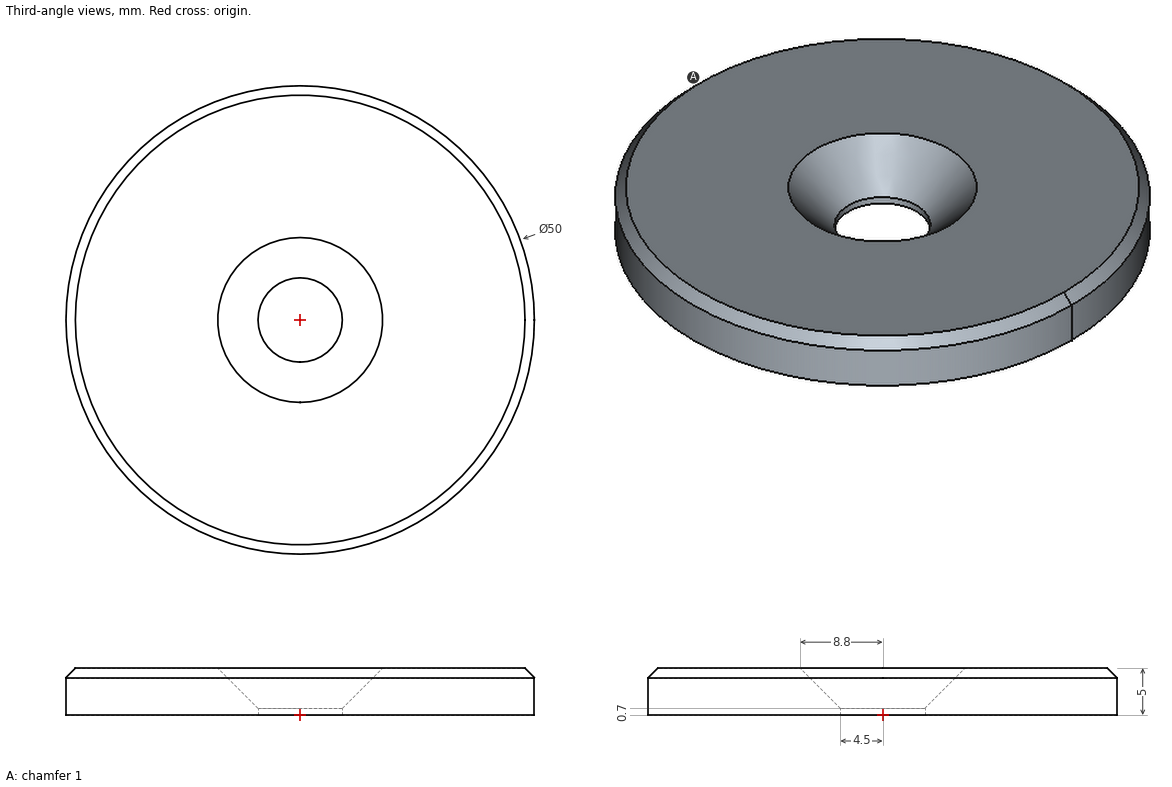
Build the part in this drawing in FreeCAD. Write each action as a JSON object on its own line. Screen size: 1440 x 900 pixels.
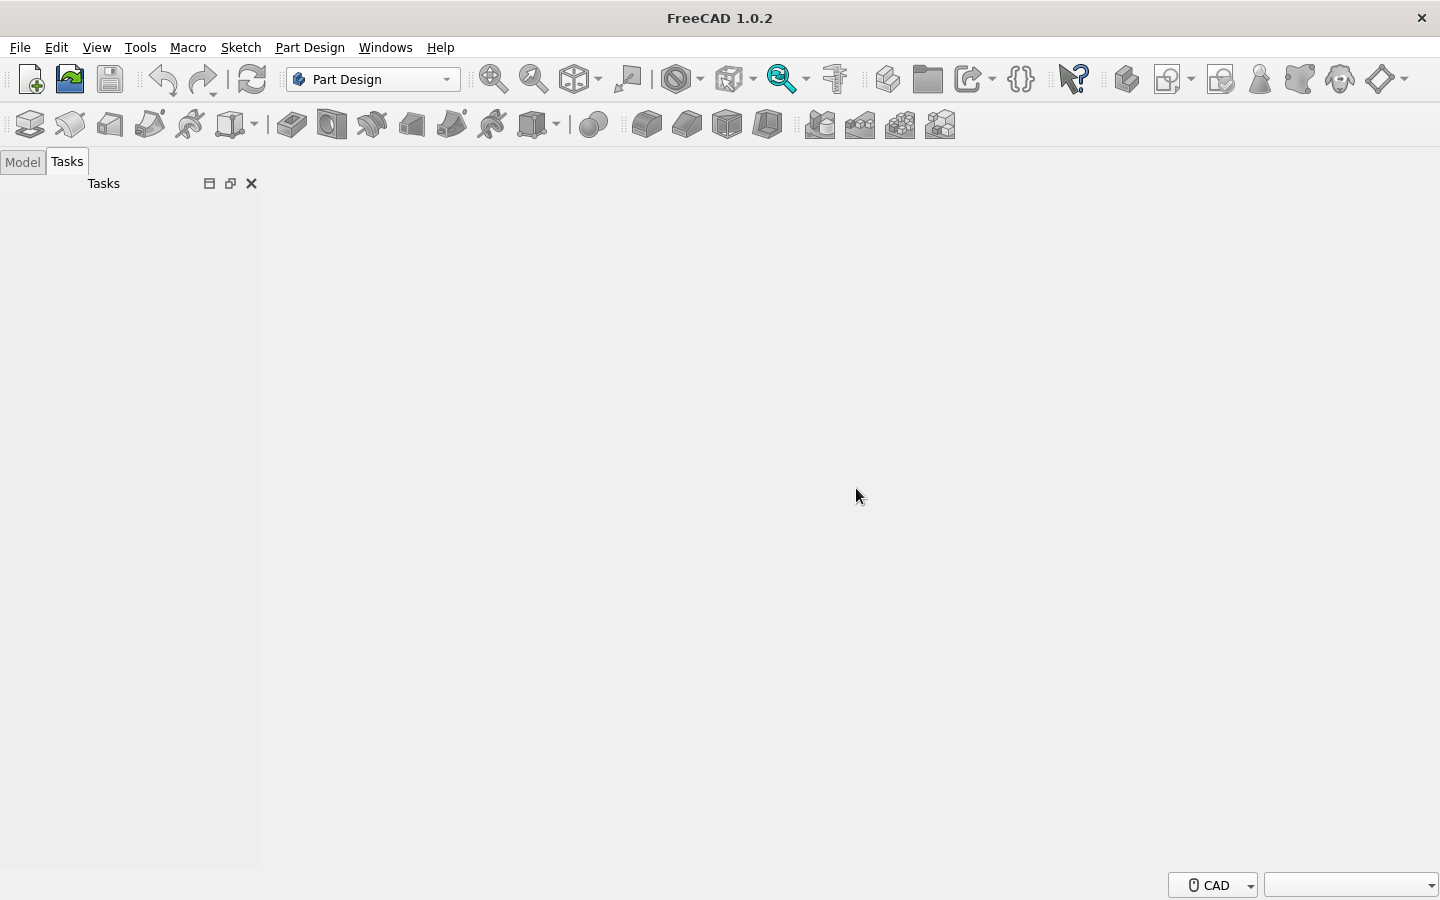
{"action": "left_click", "coordinate": [30, 80]}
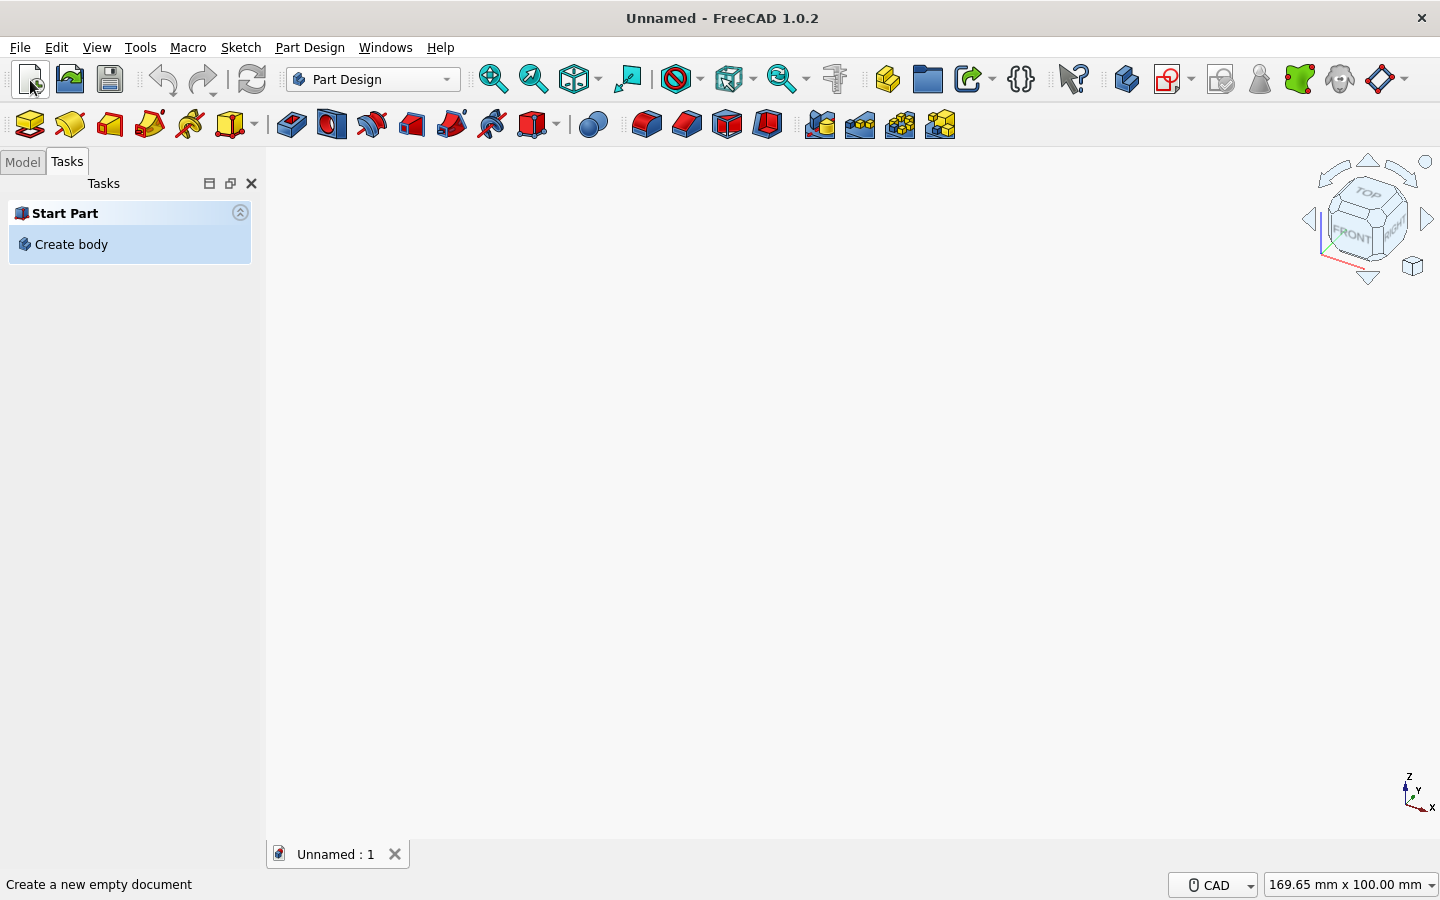
{"action": "left_click", "coordinate": [1168, 80]}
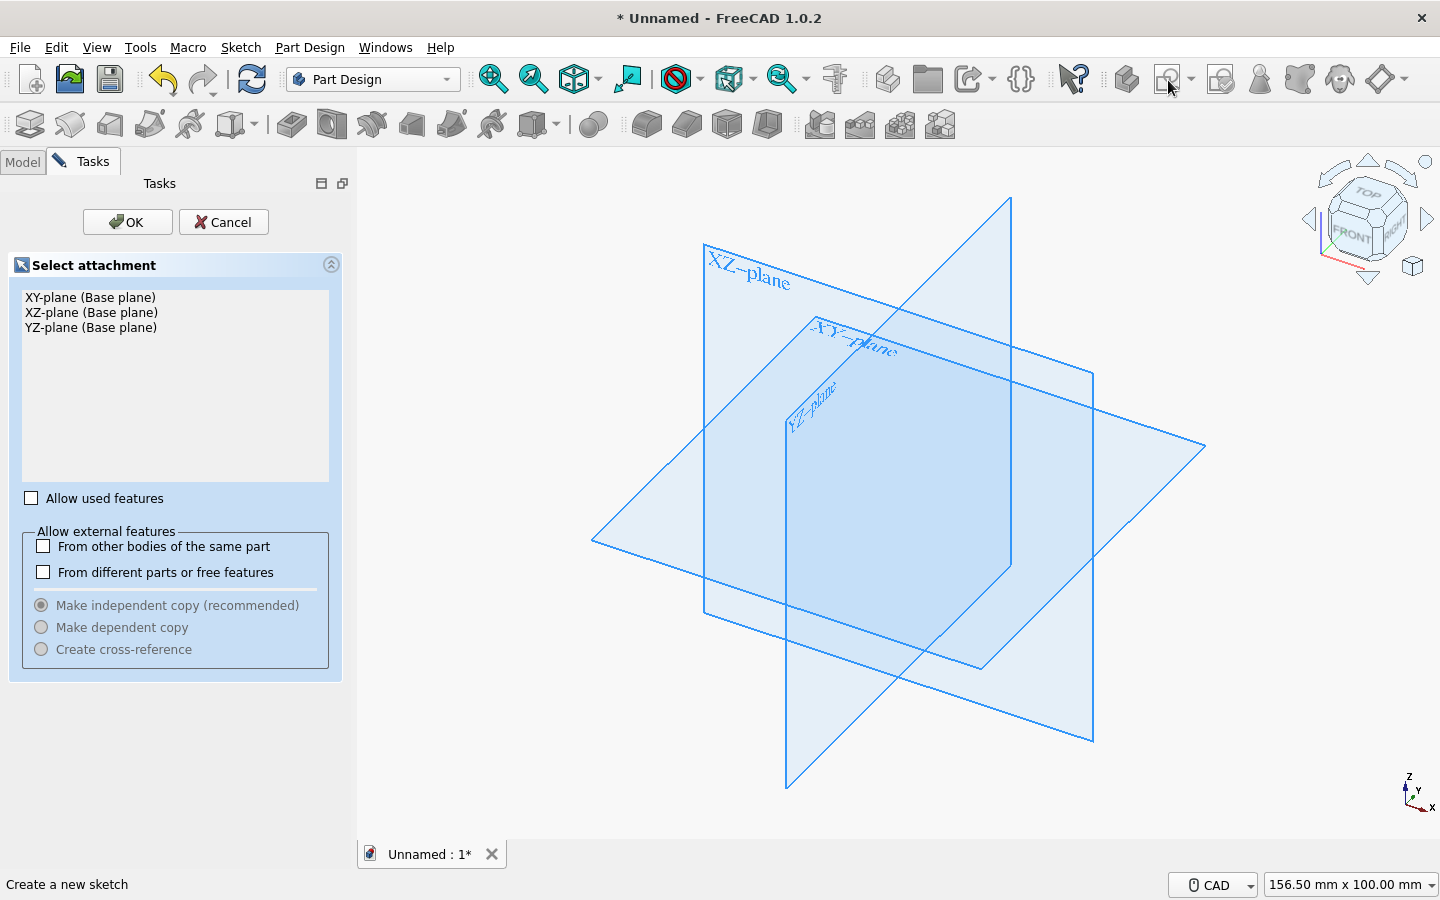
{"action": "left_click", "coordinate": [82, 298]}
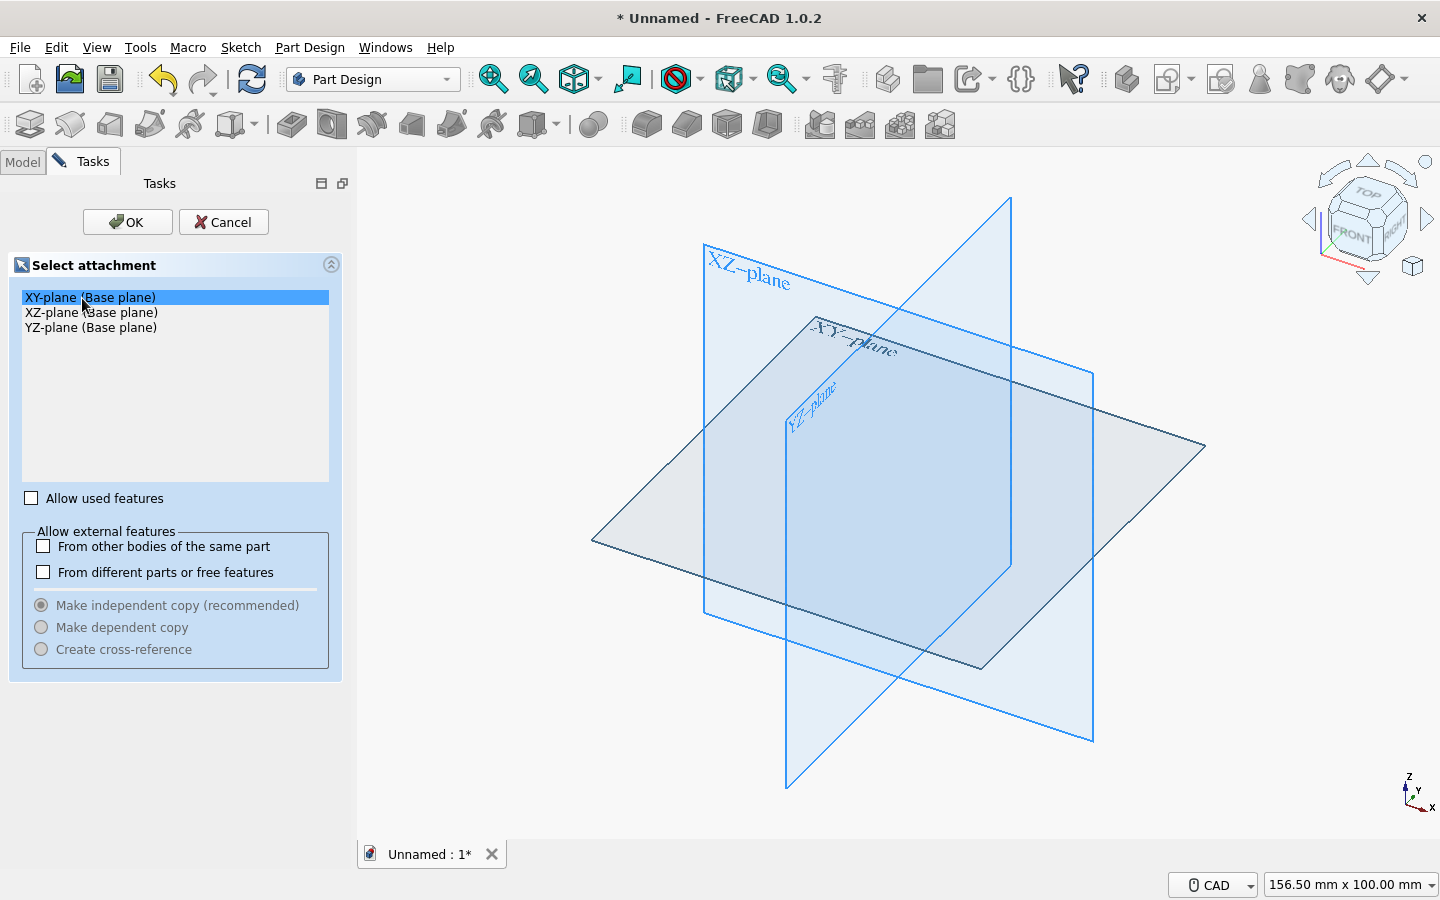
{"action": "left_click", "coordinate": [128, 222]}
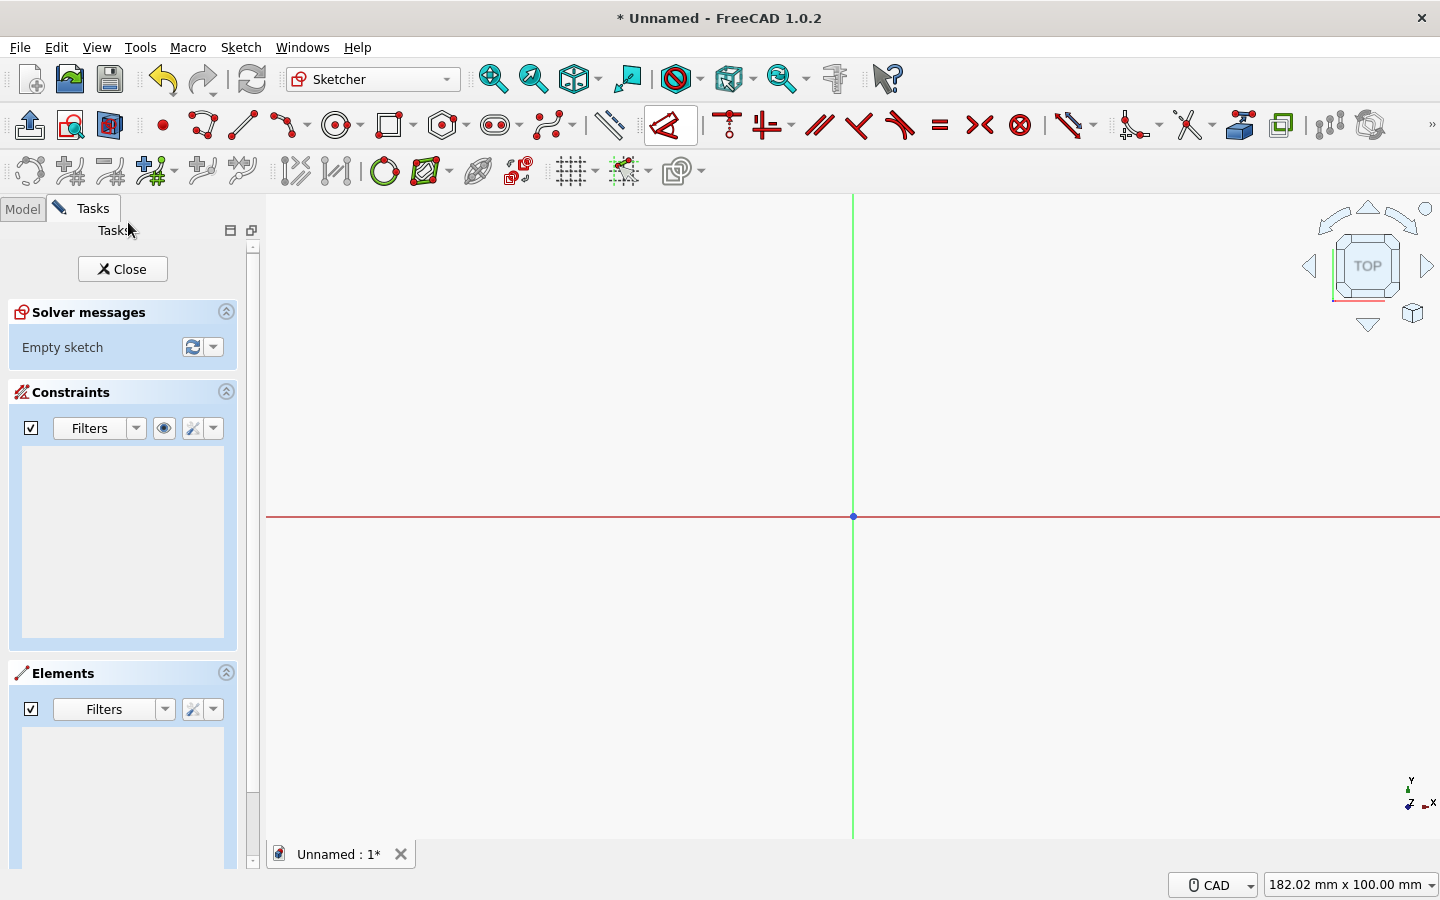
{"action": "left_click", "coordinate": [336, 126]}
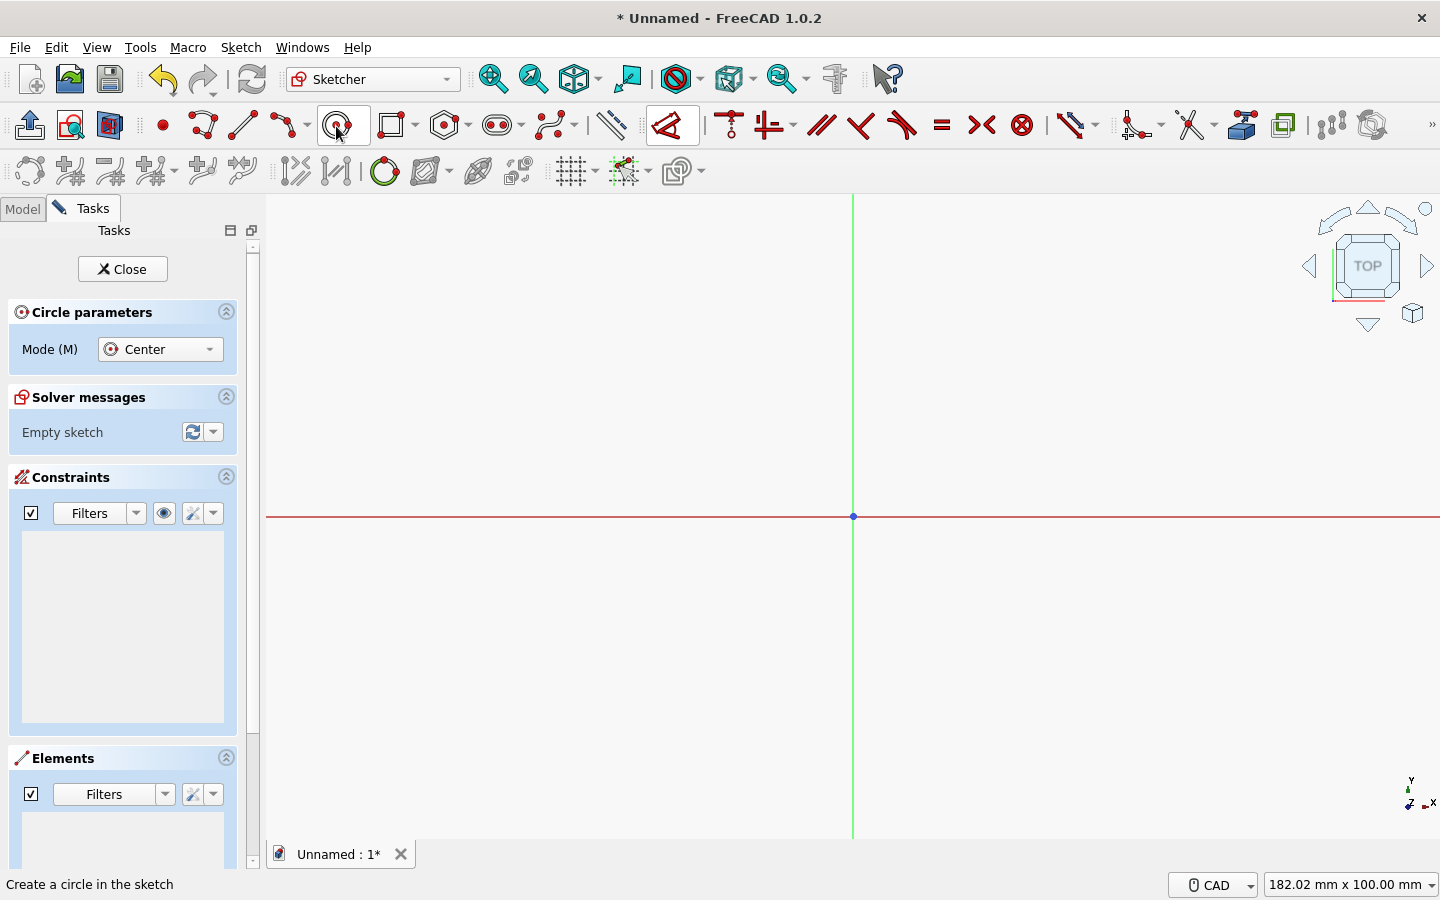
{"action": "left_click", "coordinate": [853, 516]}
{"action": "mouse_move", "coordinate": [967, 402]}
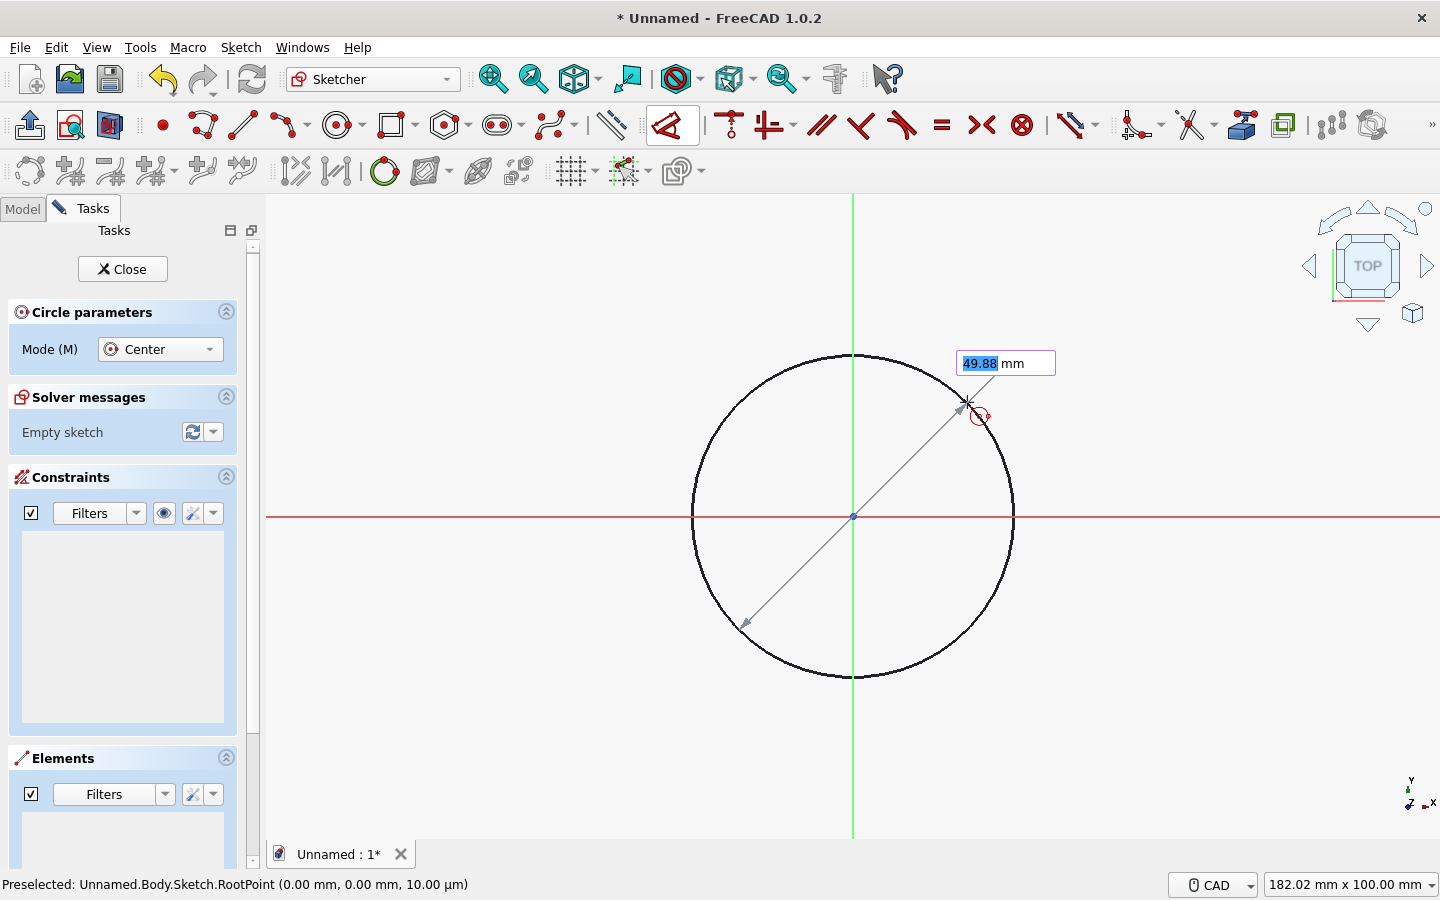
{"action": "type", "text": "50"}
{"action": "key", "text": "Return"}
{"action": "key", "text": "Escape"}